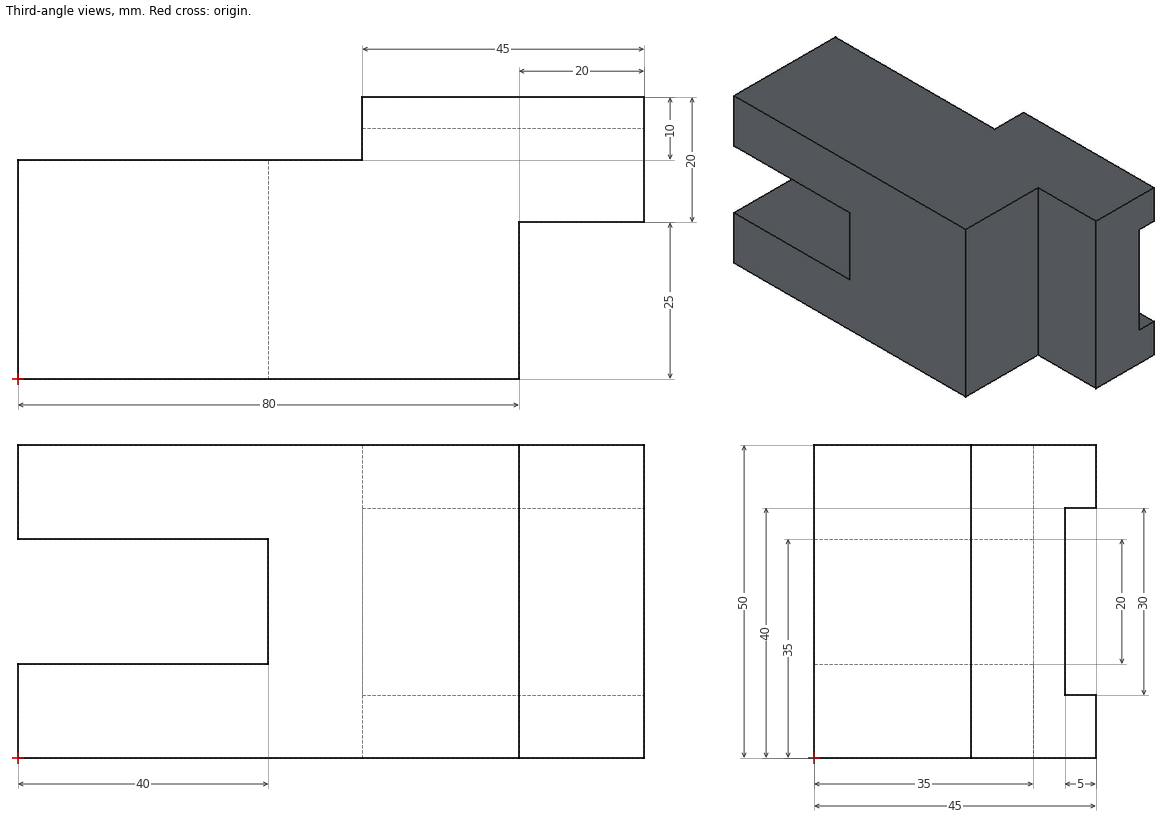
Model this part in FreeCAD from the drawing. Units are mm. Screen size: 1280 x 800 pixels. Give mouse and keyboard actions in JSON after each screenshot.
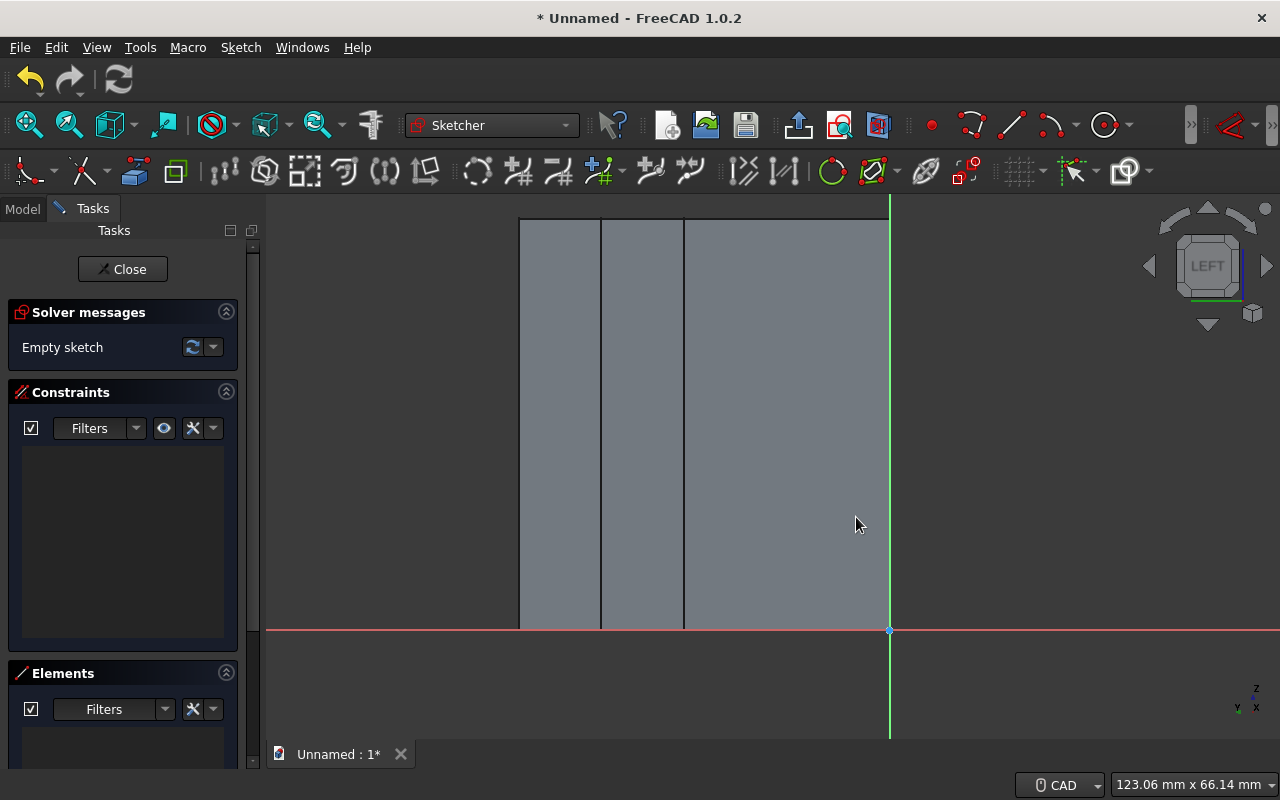
{"action": "key", "text": "g r"}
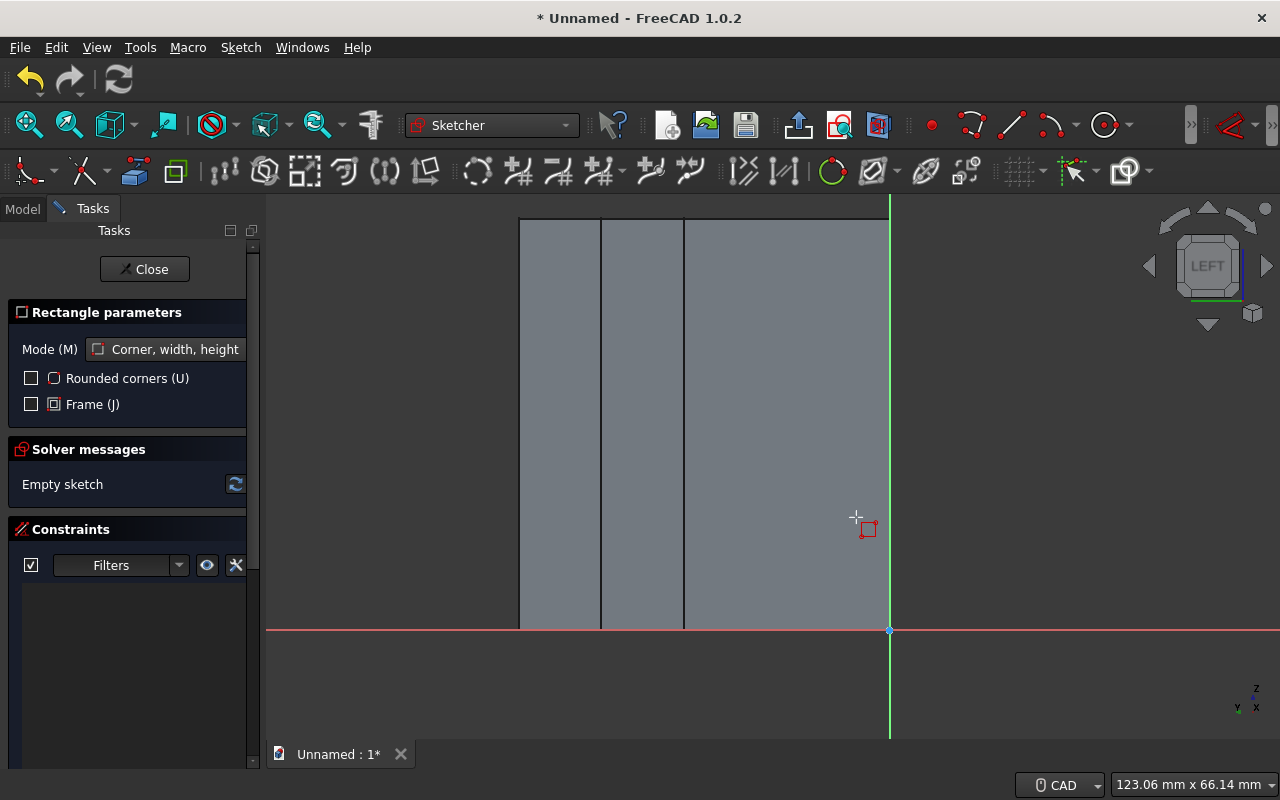
{"action": "left_click", "coordinate": [519, 301]}
{"action": "mouse_move", "coordinate": [560, 548]}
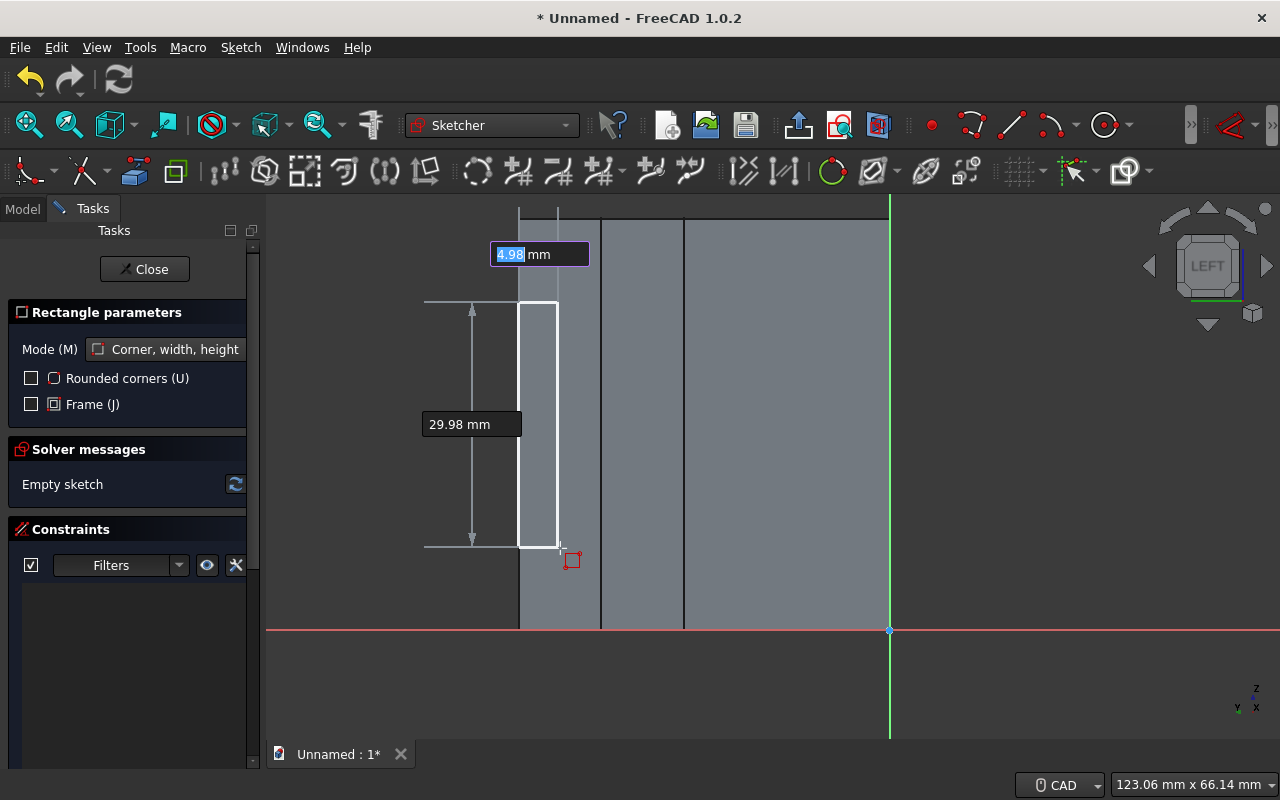
{"action": "type", "text": "5"}
{"action": "key", "text": "Tab"}
{"action": "type", "text": "30"}
{"action": "key", "text": "Return"}
{"action": "key", "text": "Escape"}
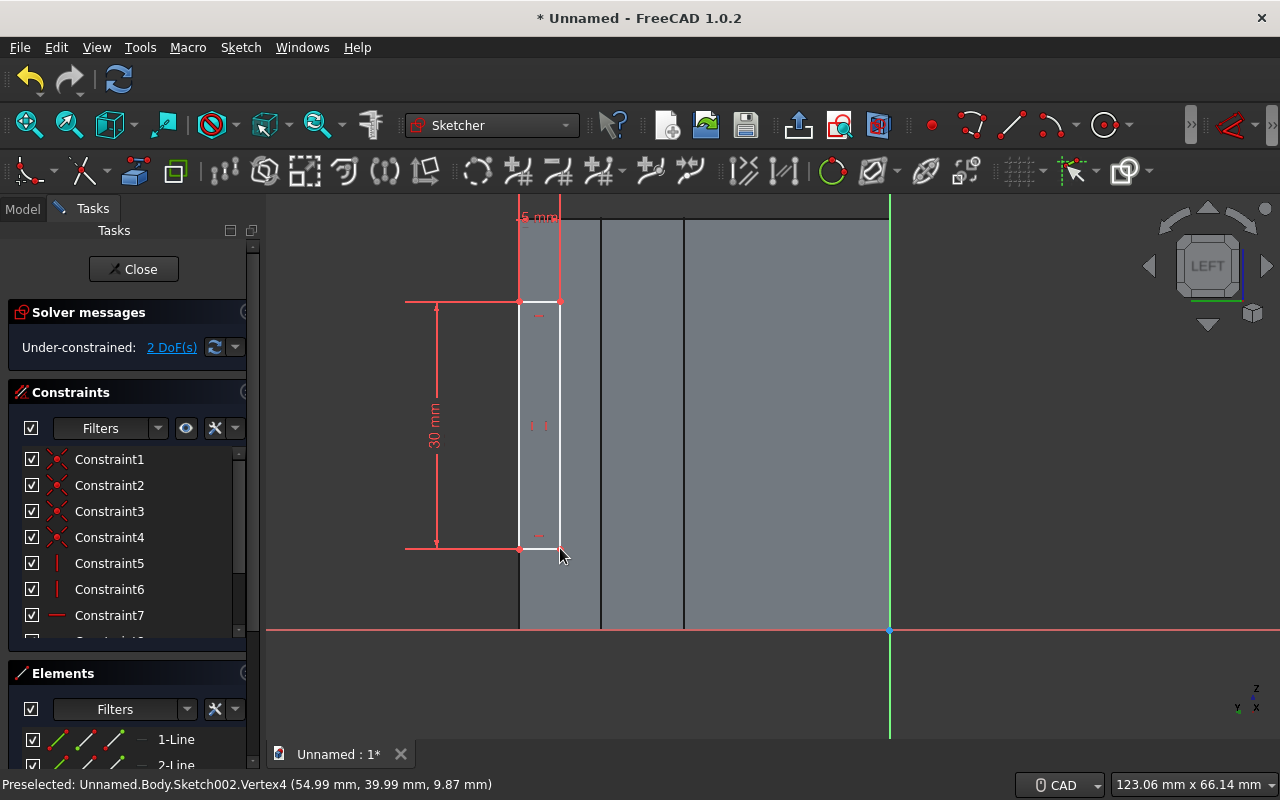
{"action": "left_click", "coordinate": [1230, 126]}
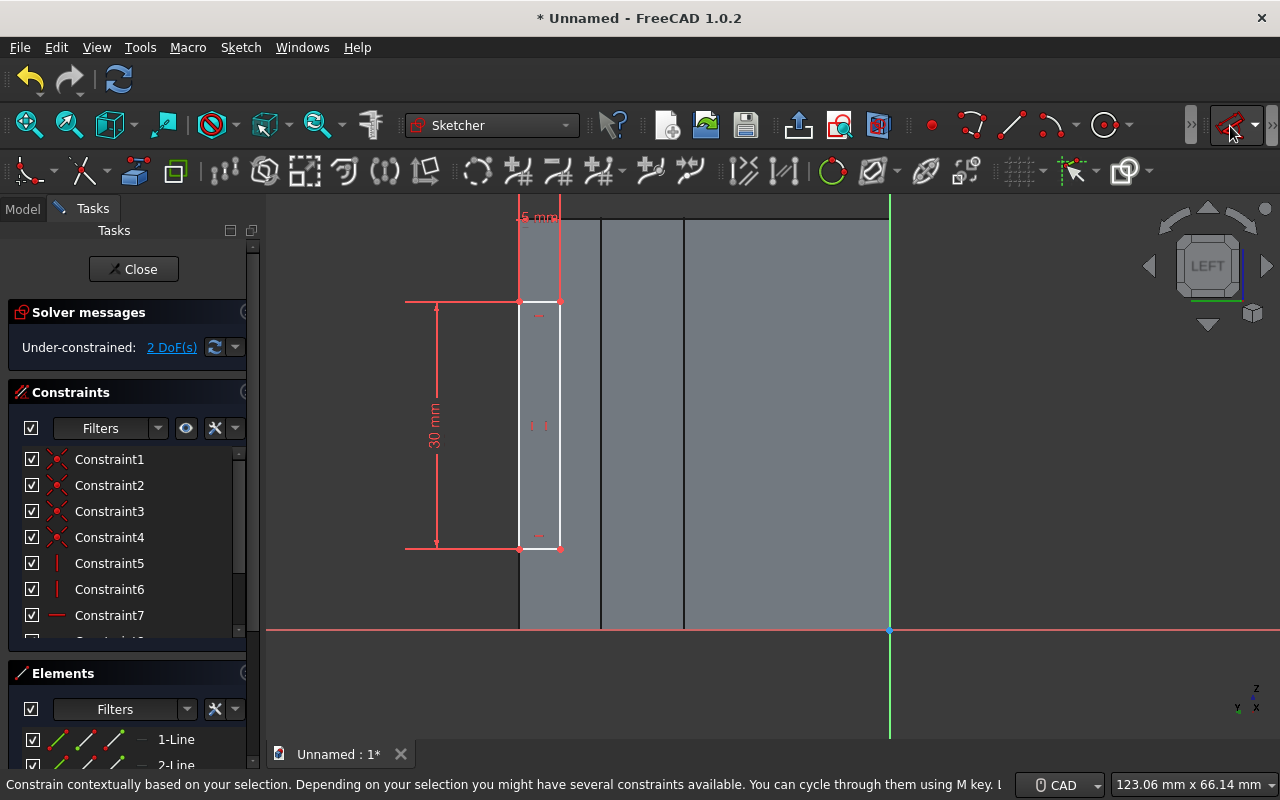
{"action": "left_click", "coordinate": [519, 302]}
{"action": "left_click", "coordinate": [704, 664]}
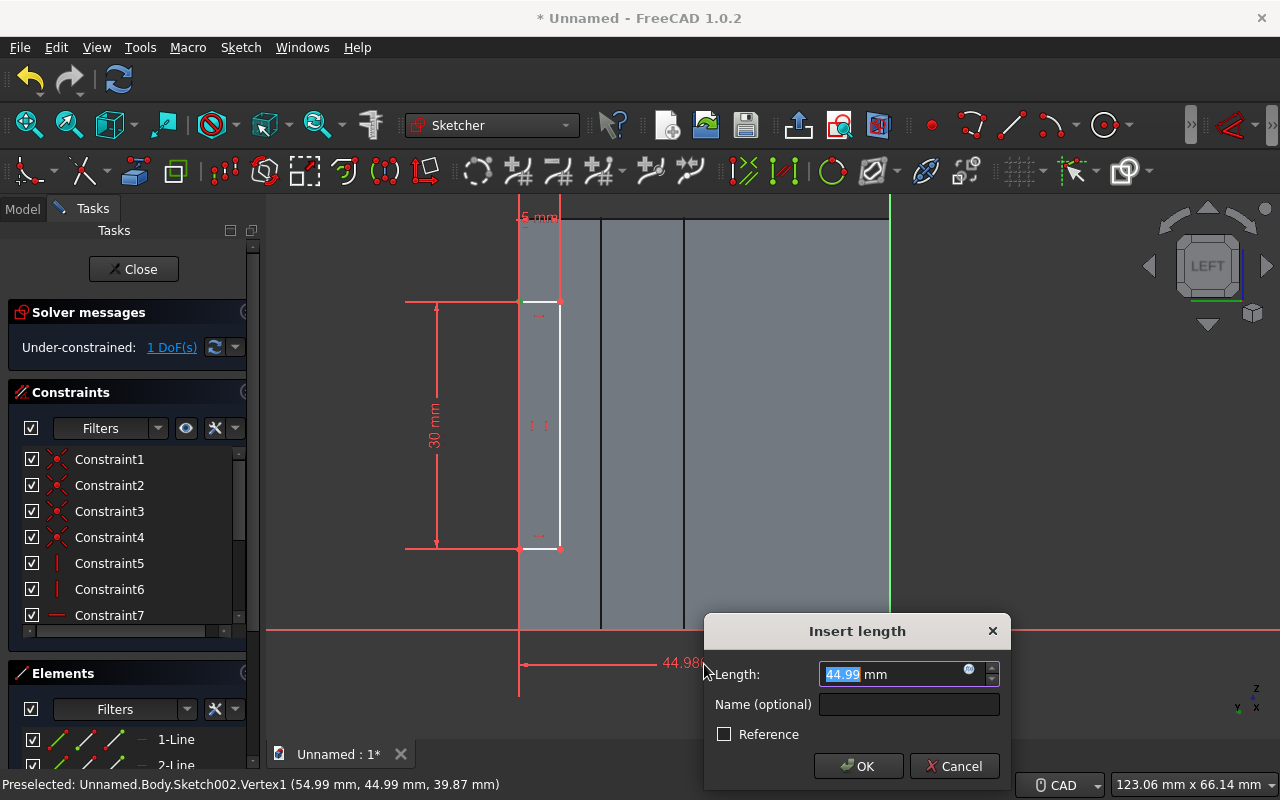
{"action": "type", "text": "45"}
{"action": "key", "text": "Return"}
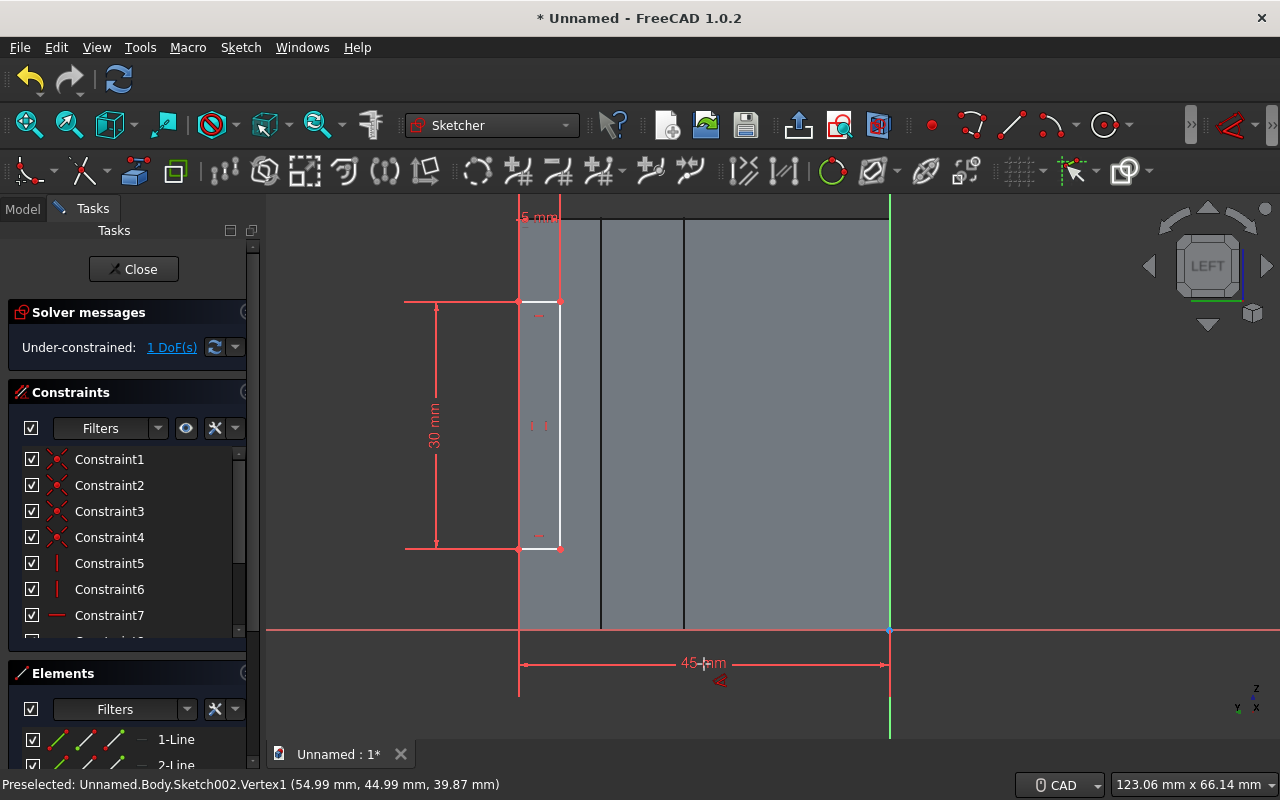
{"action": "left_click", "coordinate": [519, 302]}
{"action": "left_click", "coordinate": [924, 466]}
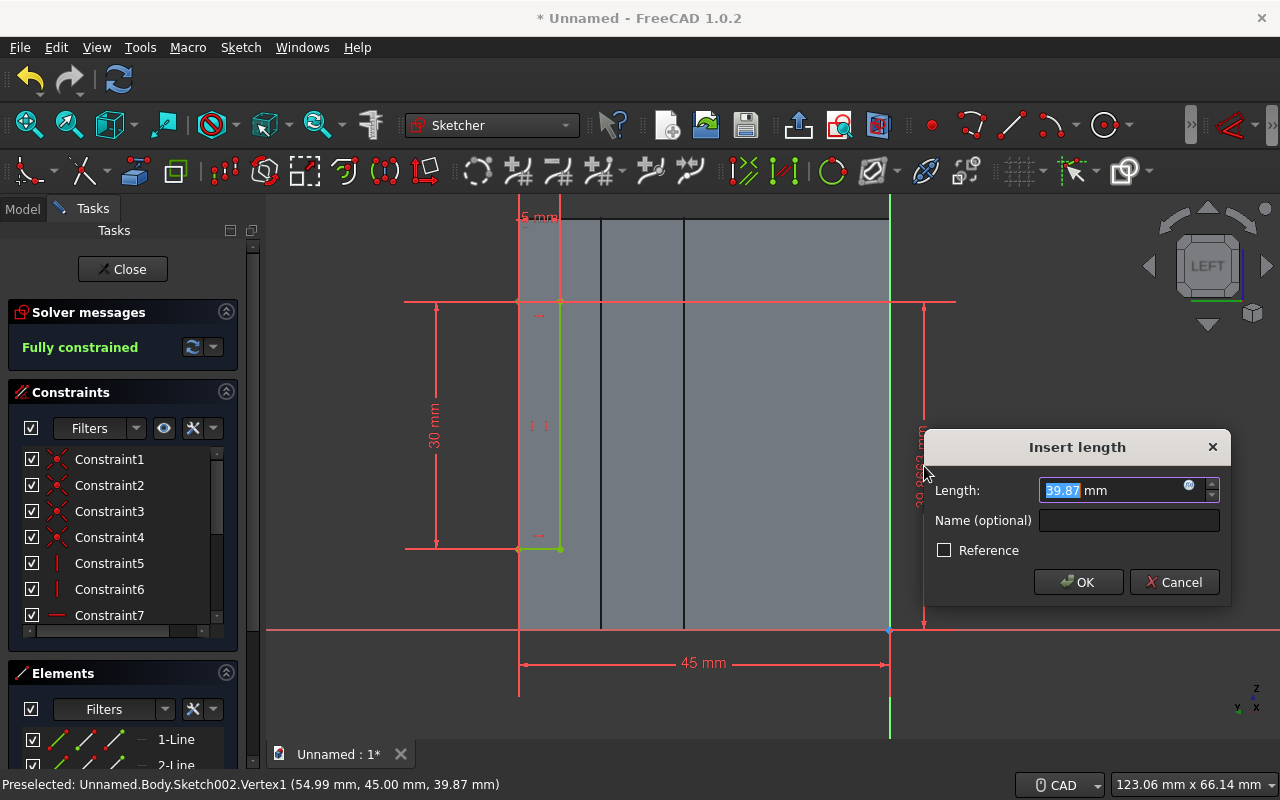
{"action": "type", "text": "40"}
{"action": "key", "text": "Return"}
{"action": "key", "text": "Escape"}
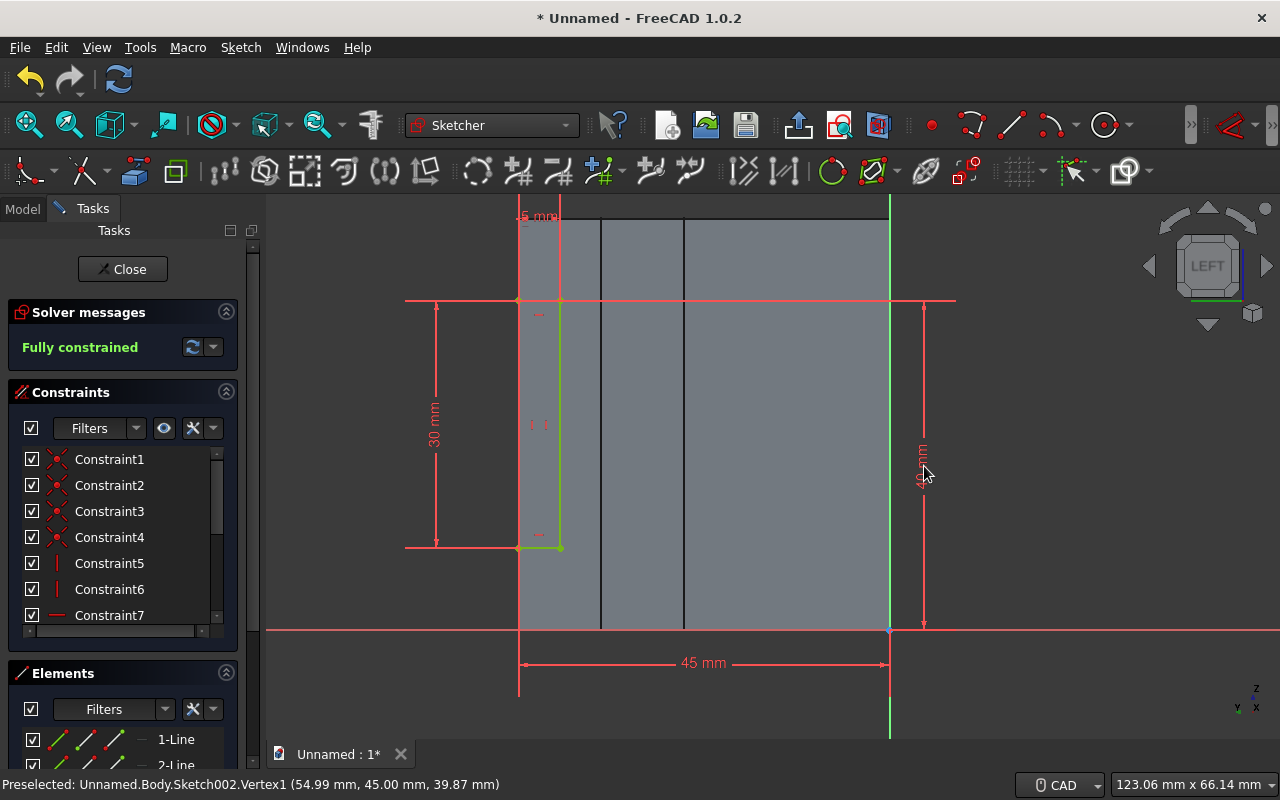
{"action": "left_click", "coordinate": [123, 269]}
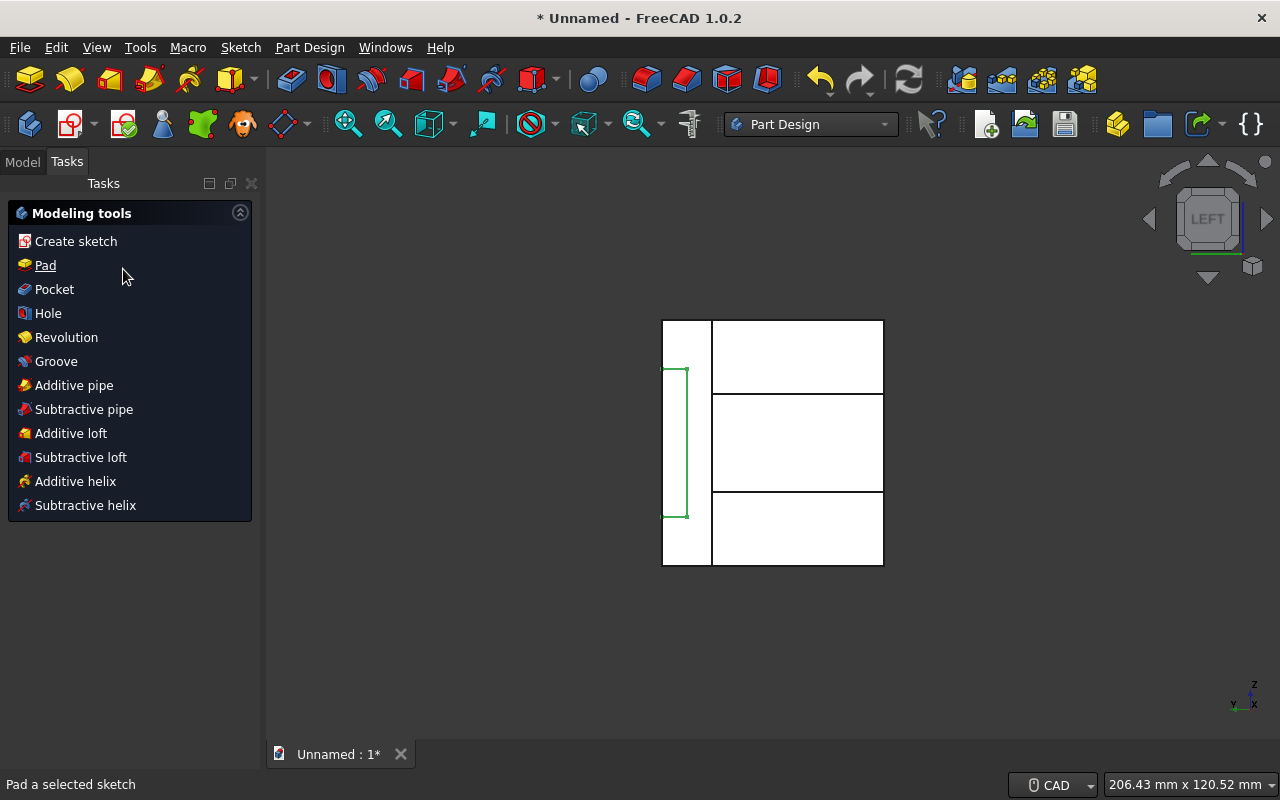
{"action": "left_click", "coordinate": [292, 80]}